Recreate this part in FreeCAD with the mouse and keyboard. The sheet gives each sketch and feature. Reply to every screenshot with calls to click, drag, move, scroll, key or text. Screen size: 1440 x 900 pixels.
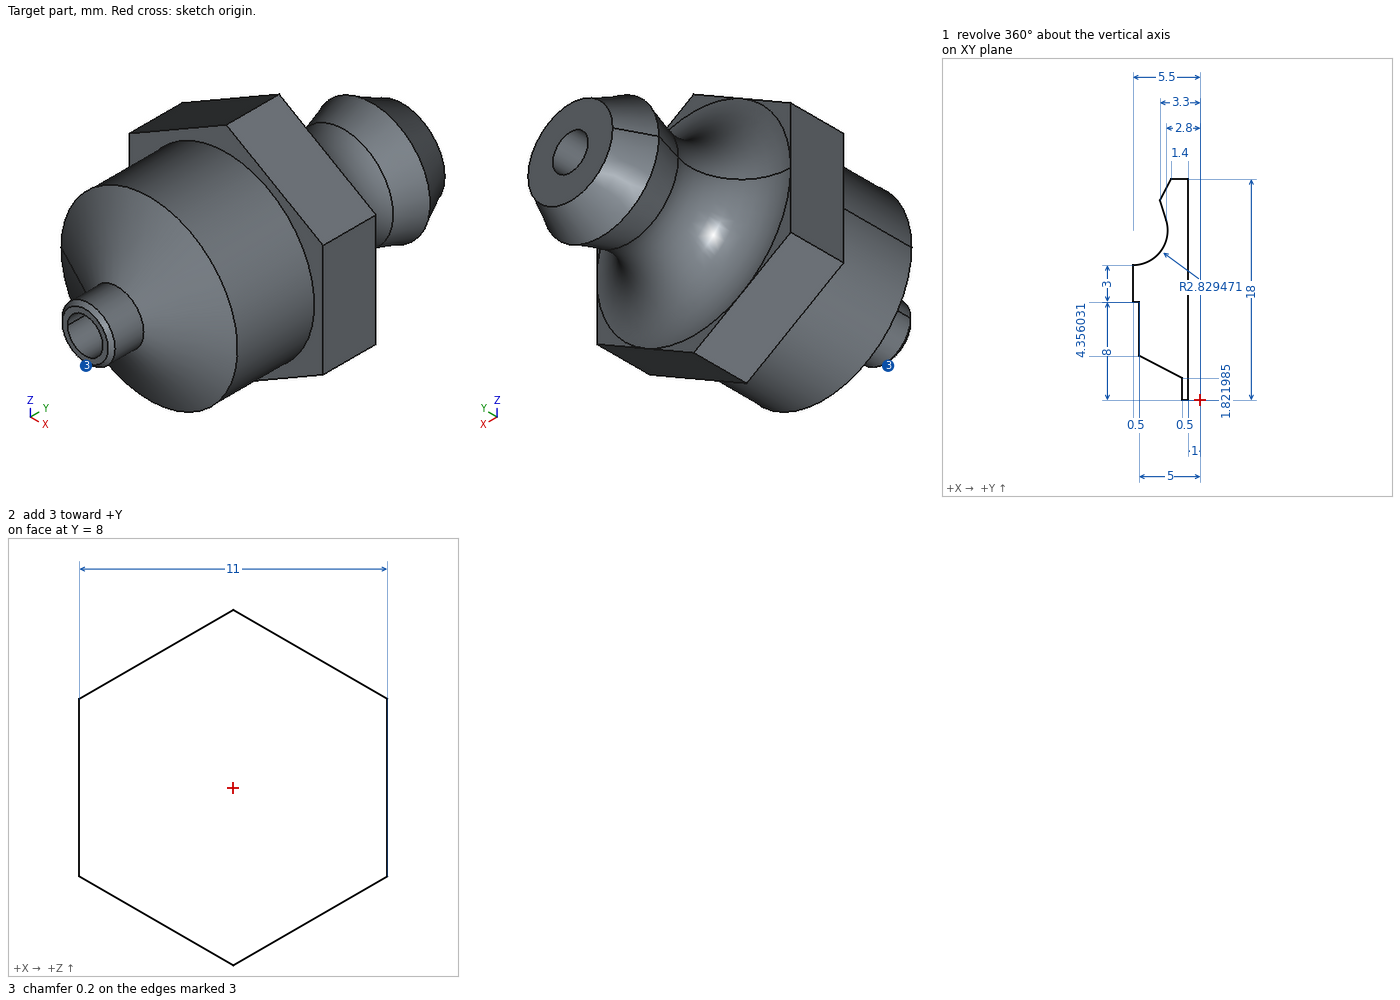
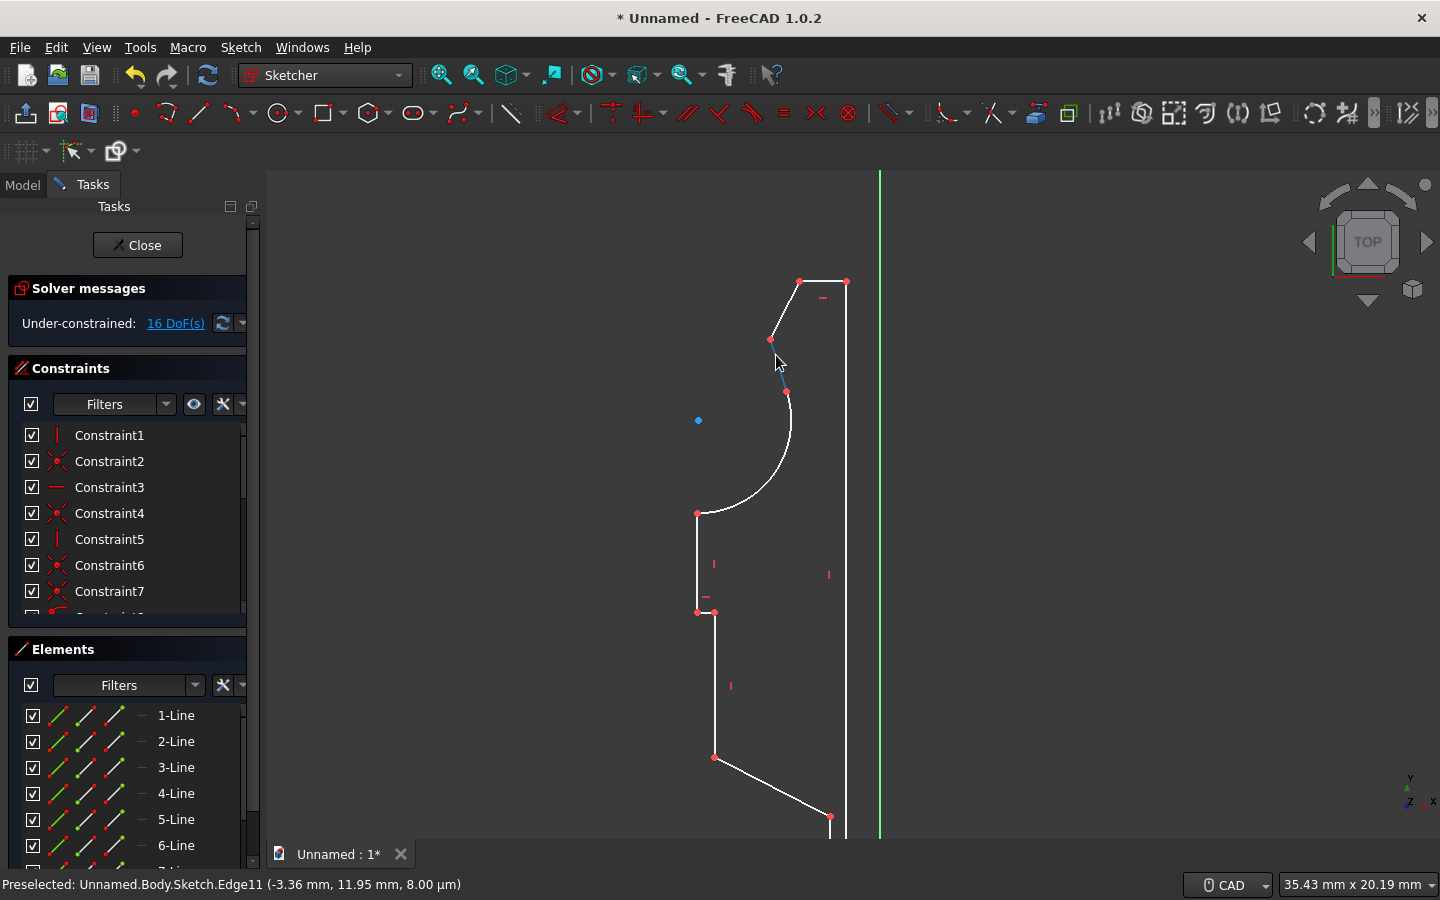
click(775, 355)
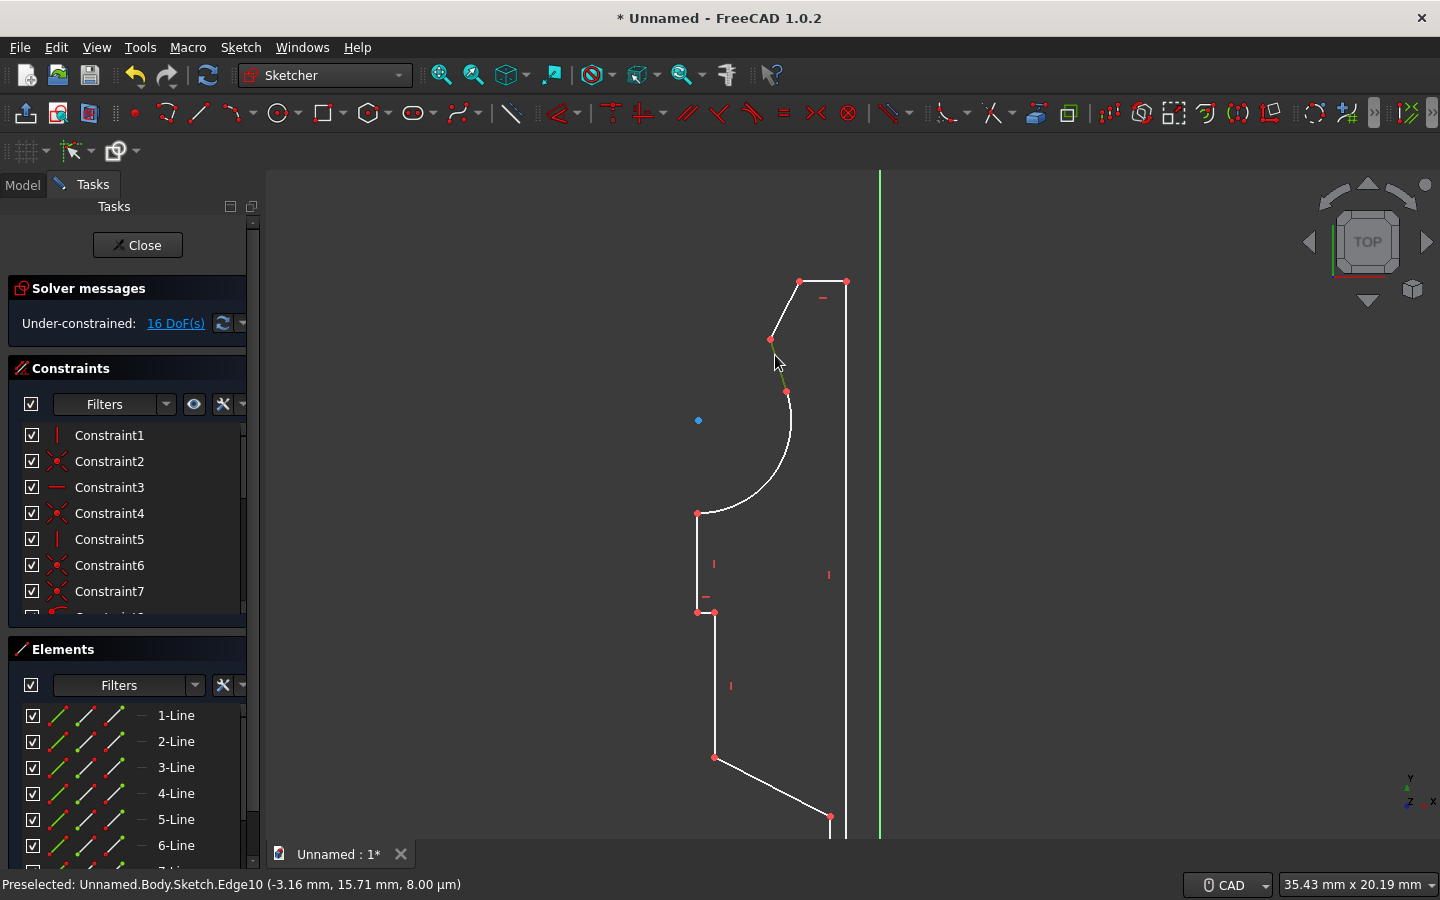
click(748, 499)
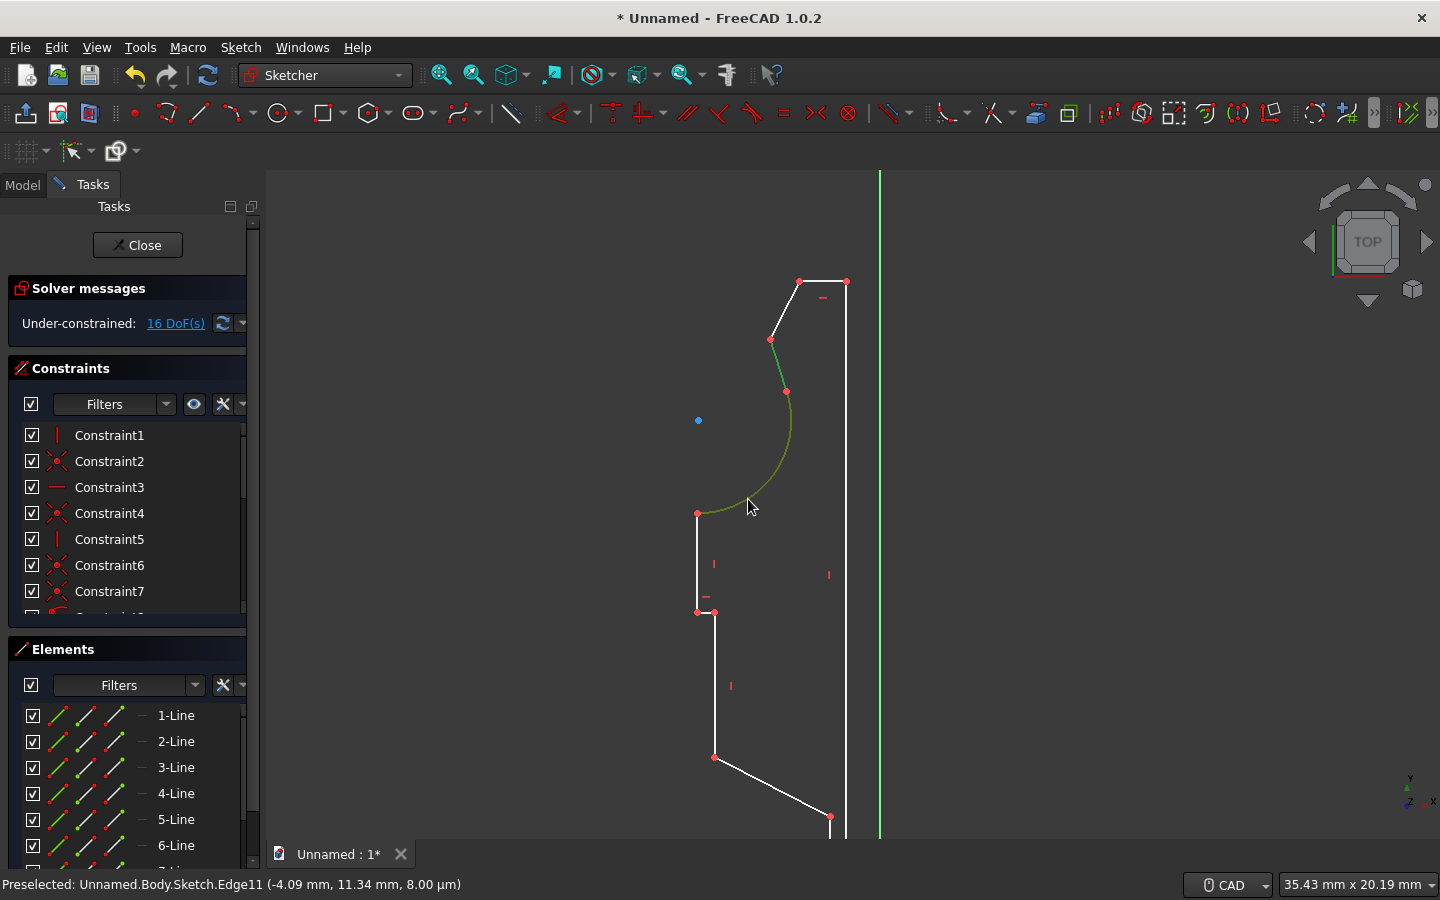
click(752, 114)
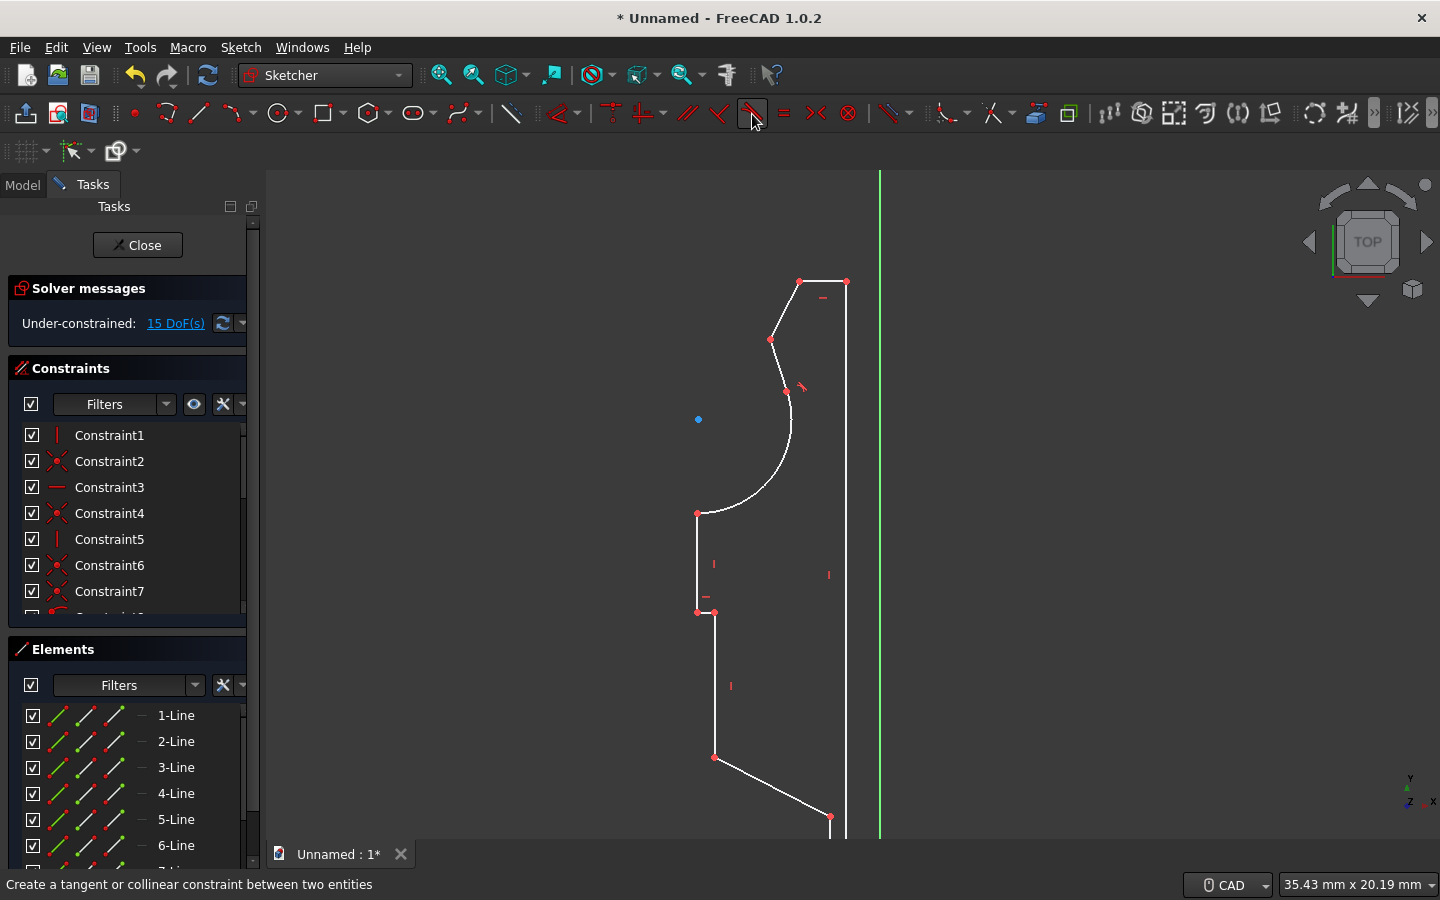
scroll(776, 354, down, 2)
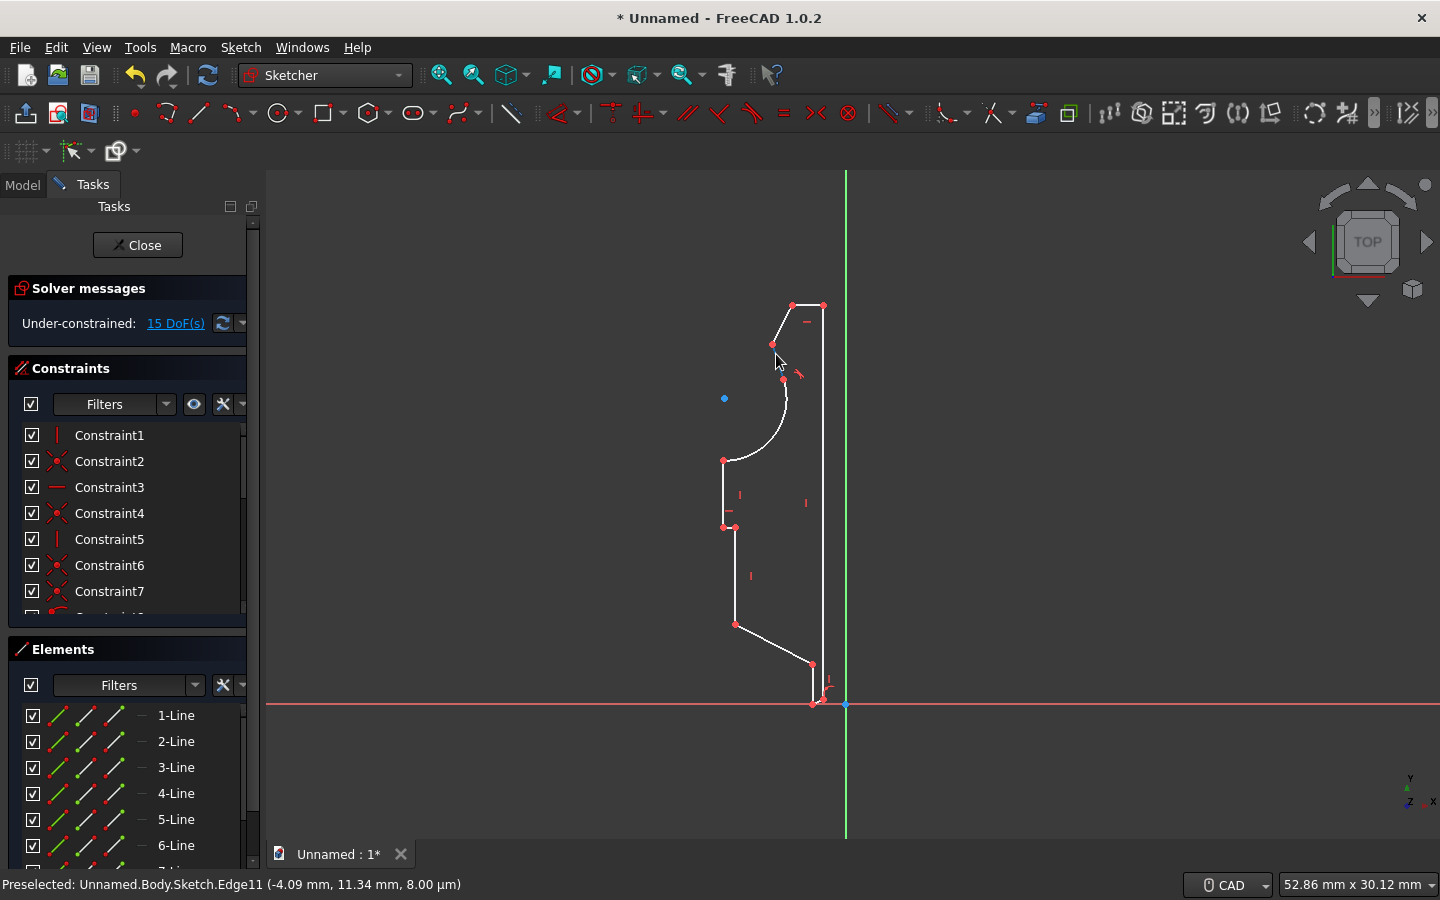
scroll(818, 702, up, 5)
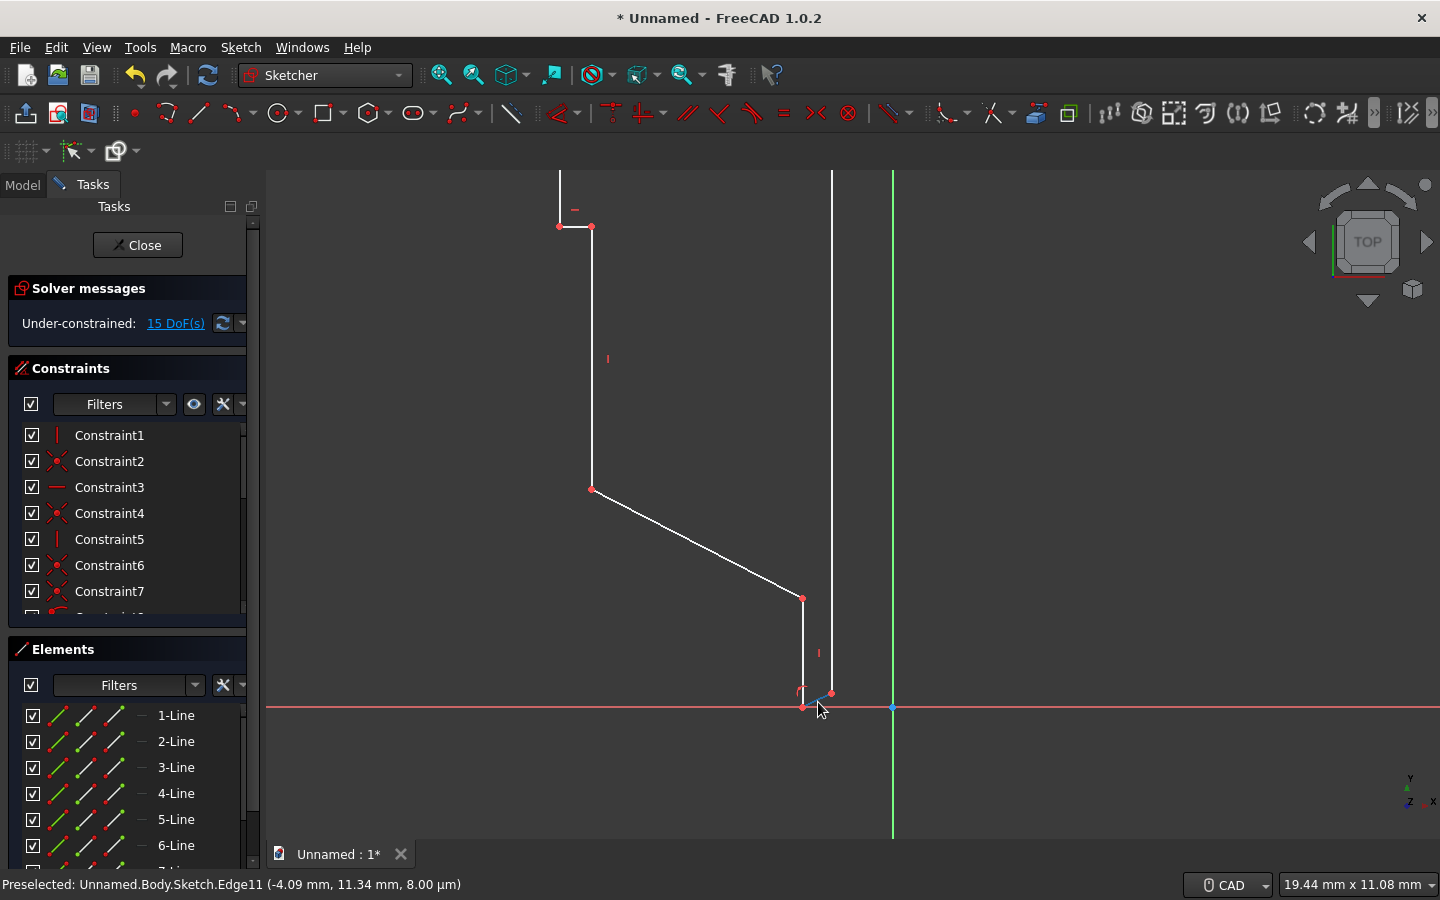
click(817, 700)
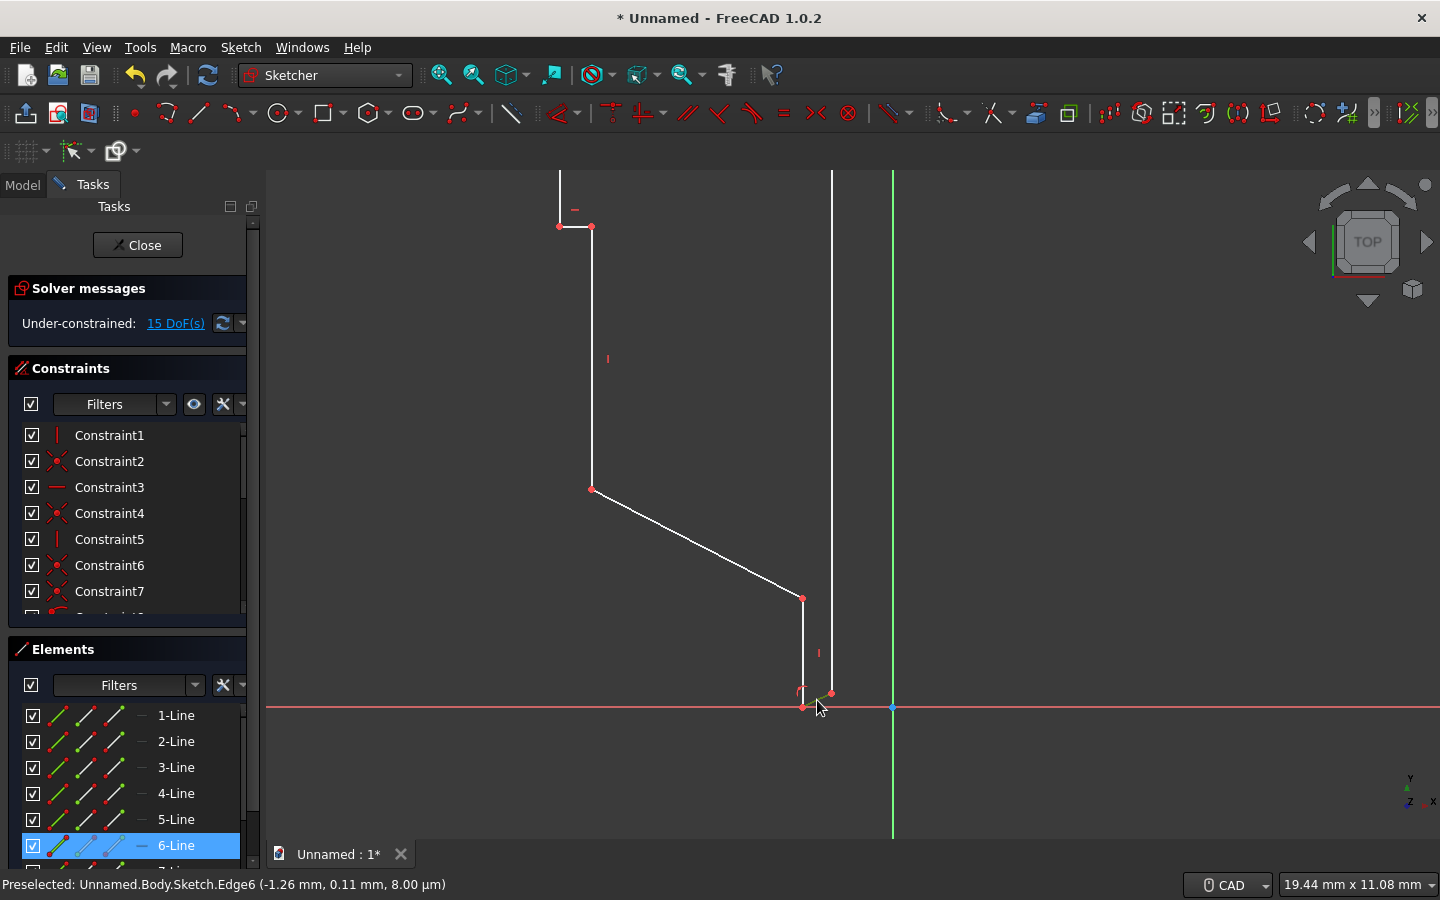
click(666, 114)